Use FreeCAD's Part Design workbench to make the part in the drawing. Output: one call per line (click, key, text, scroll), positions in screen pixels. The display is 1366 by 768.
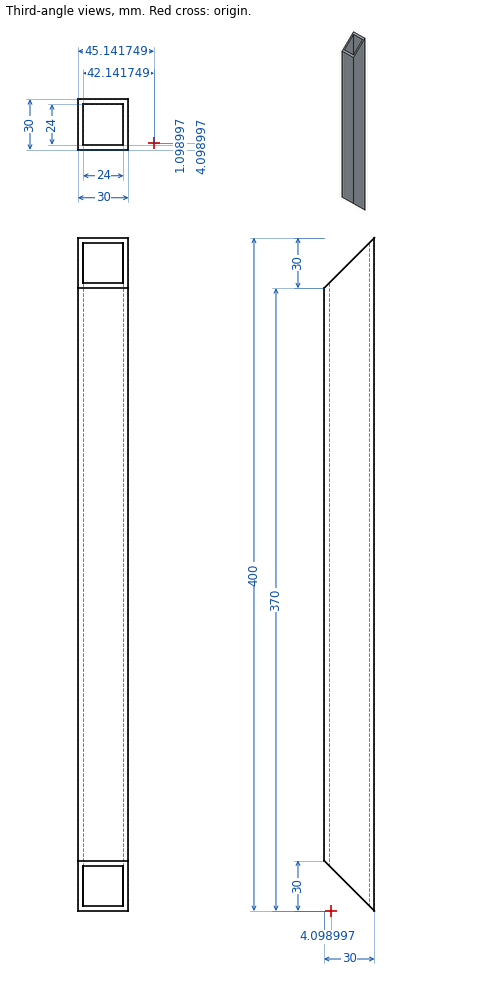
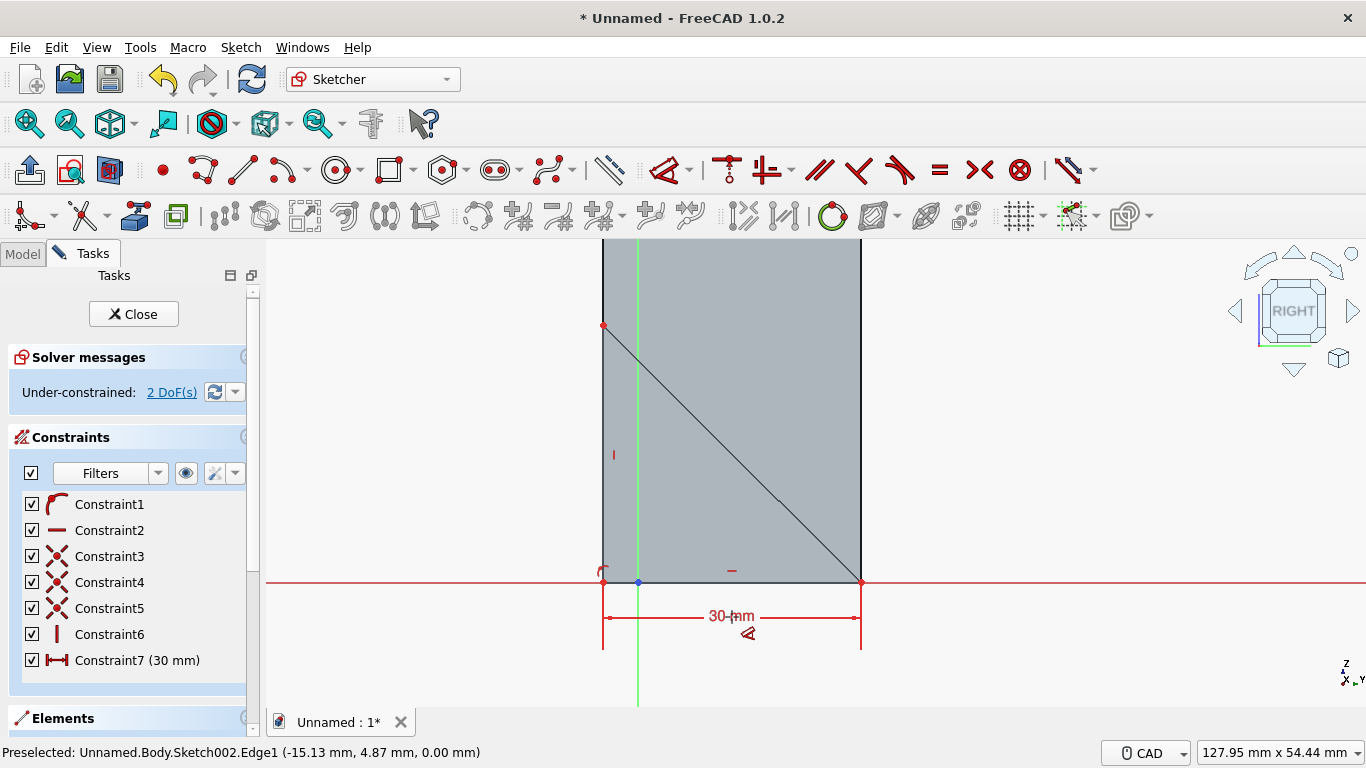
click(603, 403)
click(569, 454)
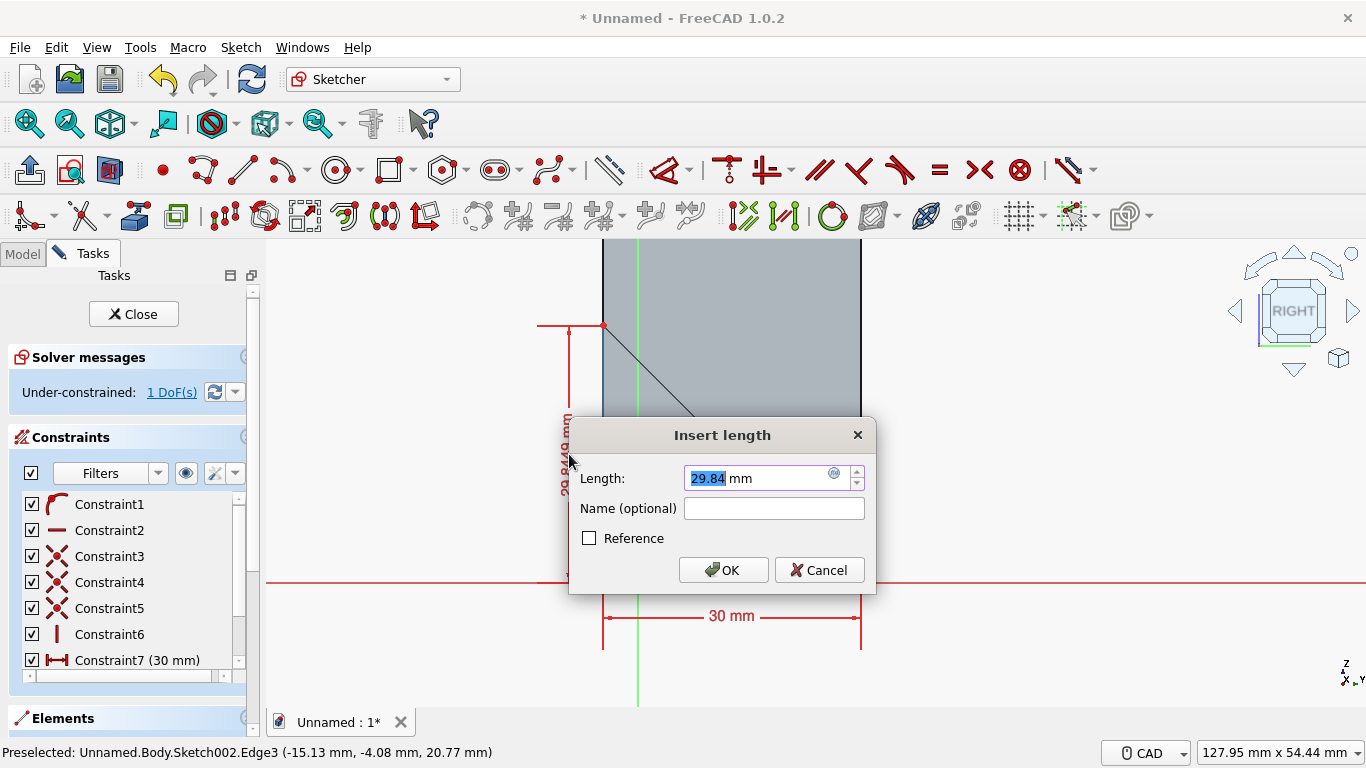
text(30)
key(Return)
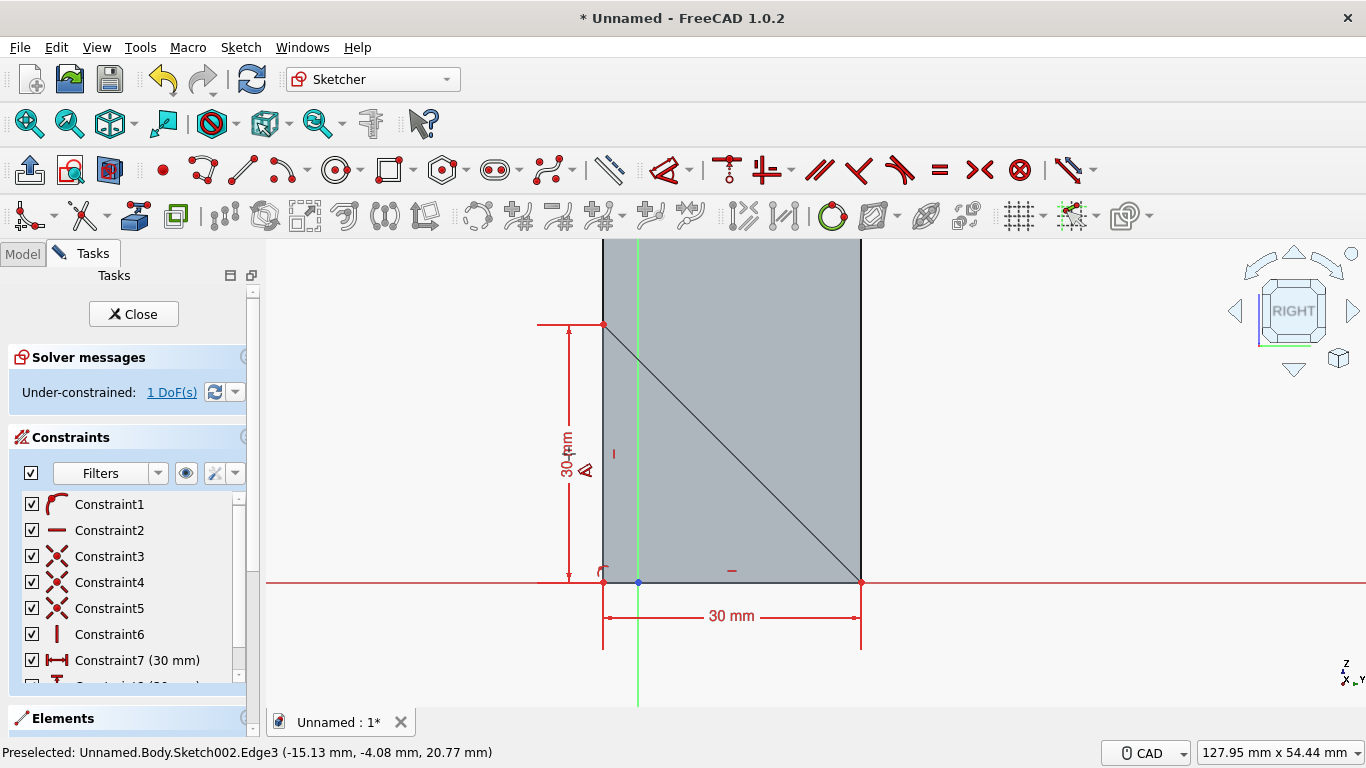
click(603, 583)
click(621, 617)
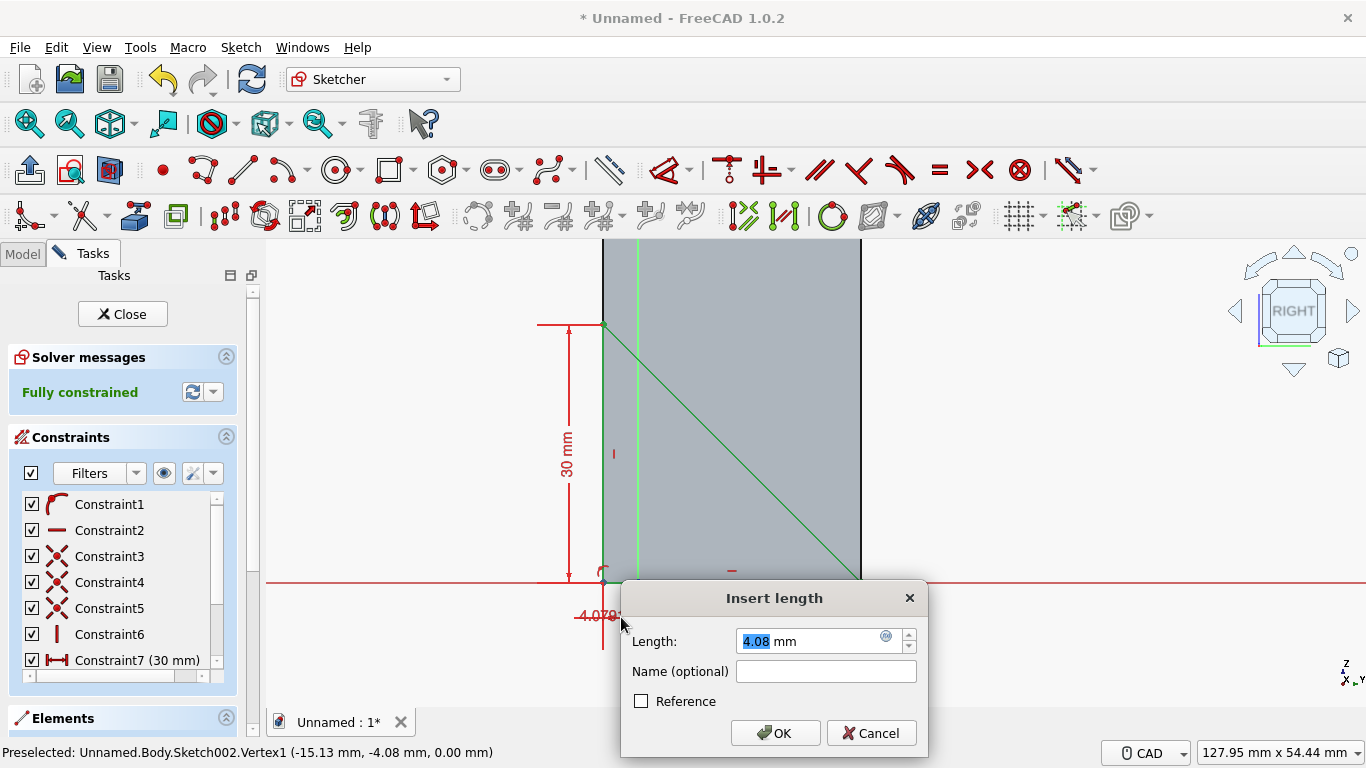
text(4.098997)
key(Return)
key(Escape)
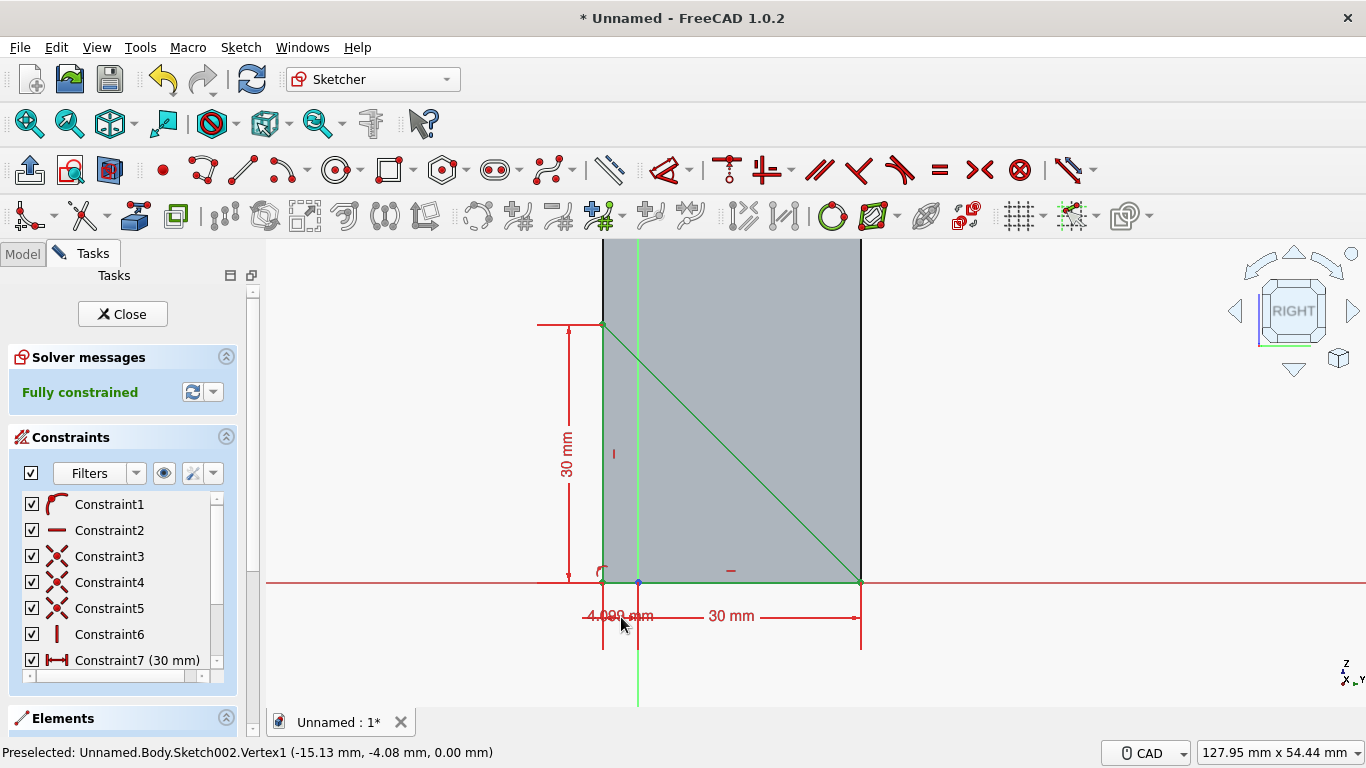
click(123, 314)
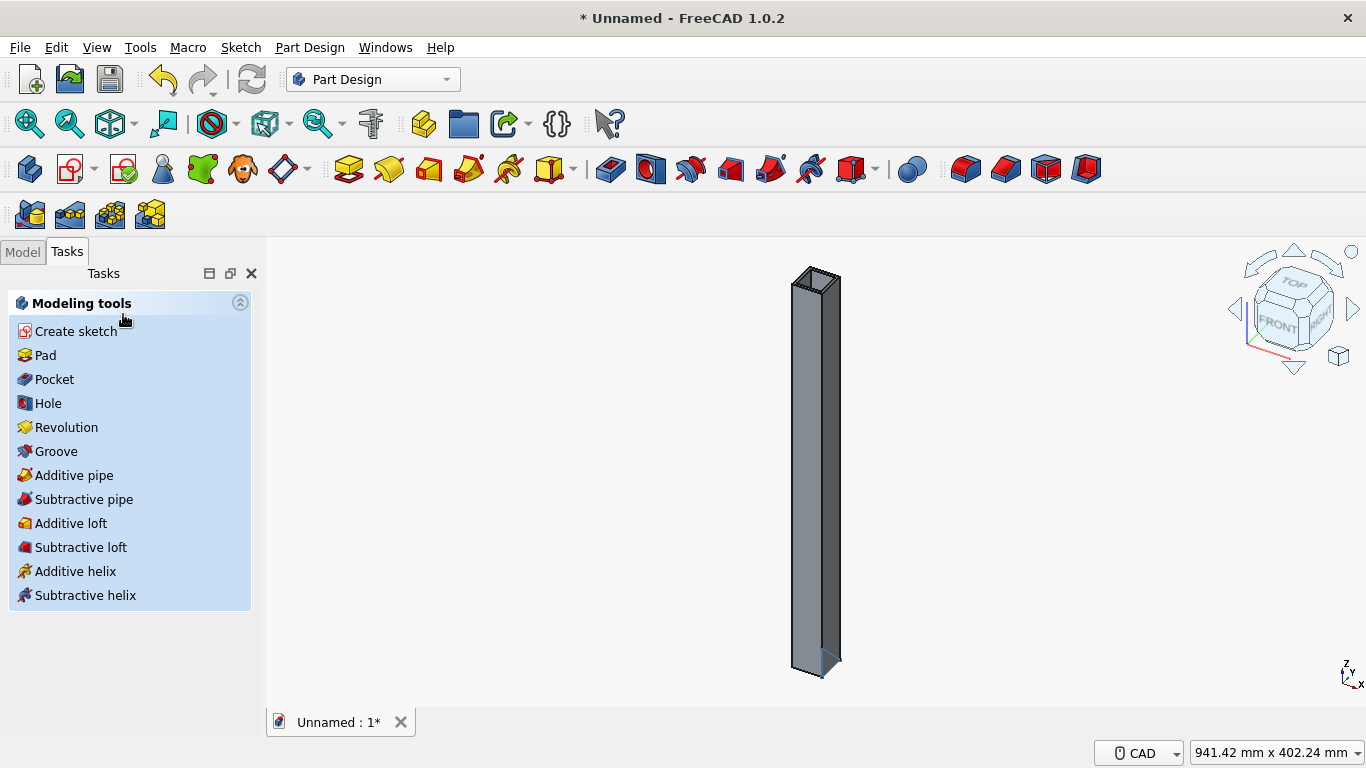
click(612, 170)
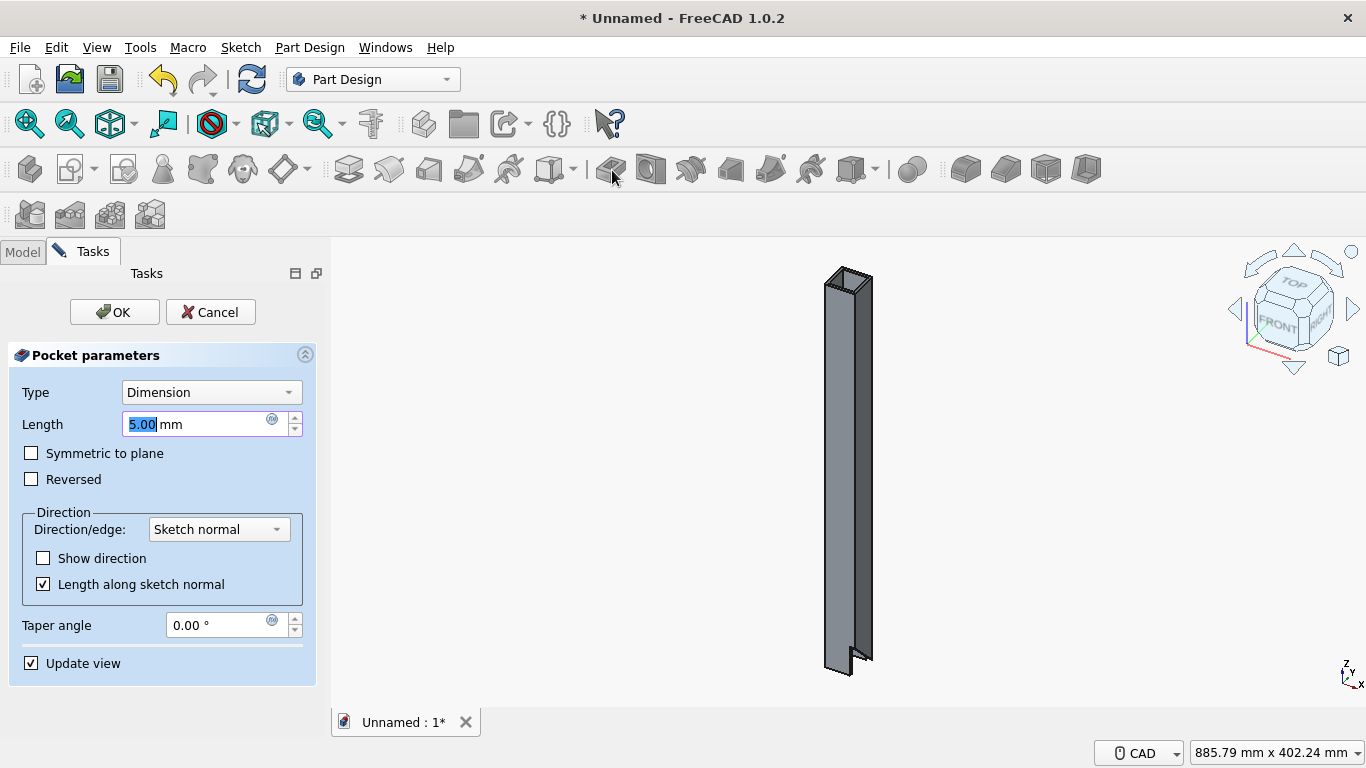
click(212, 392)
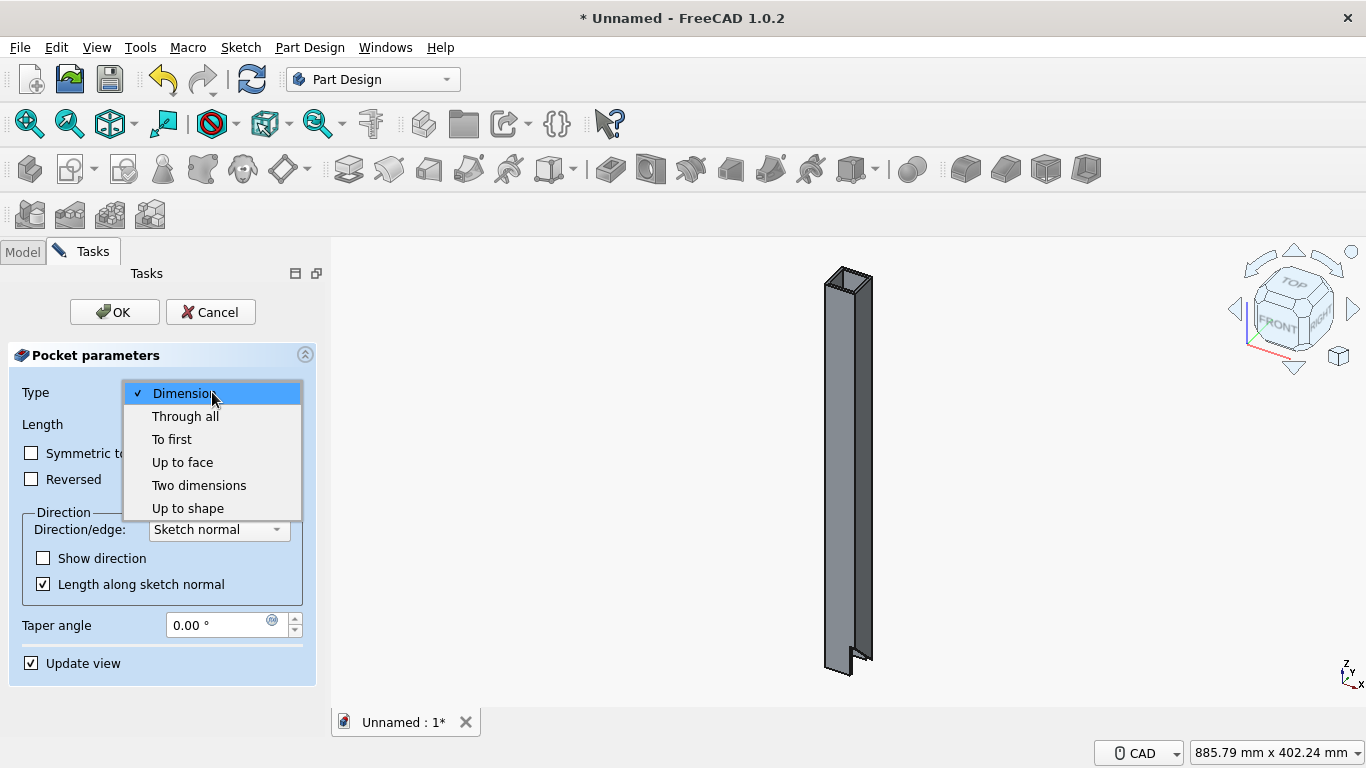
click(212, 416)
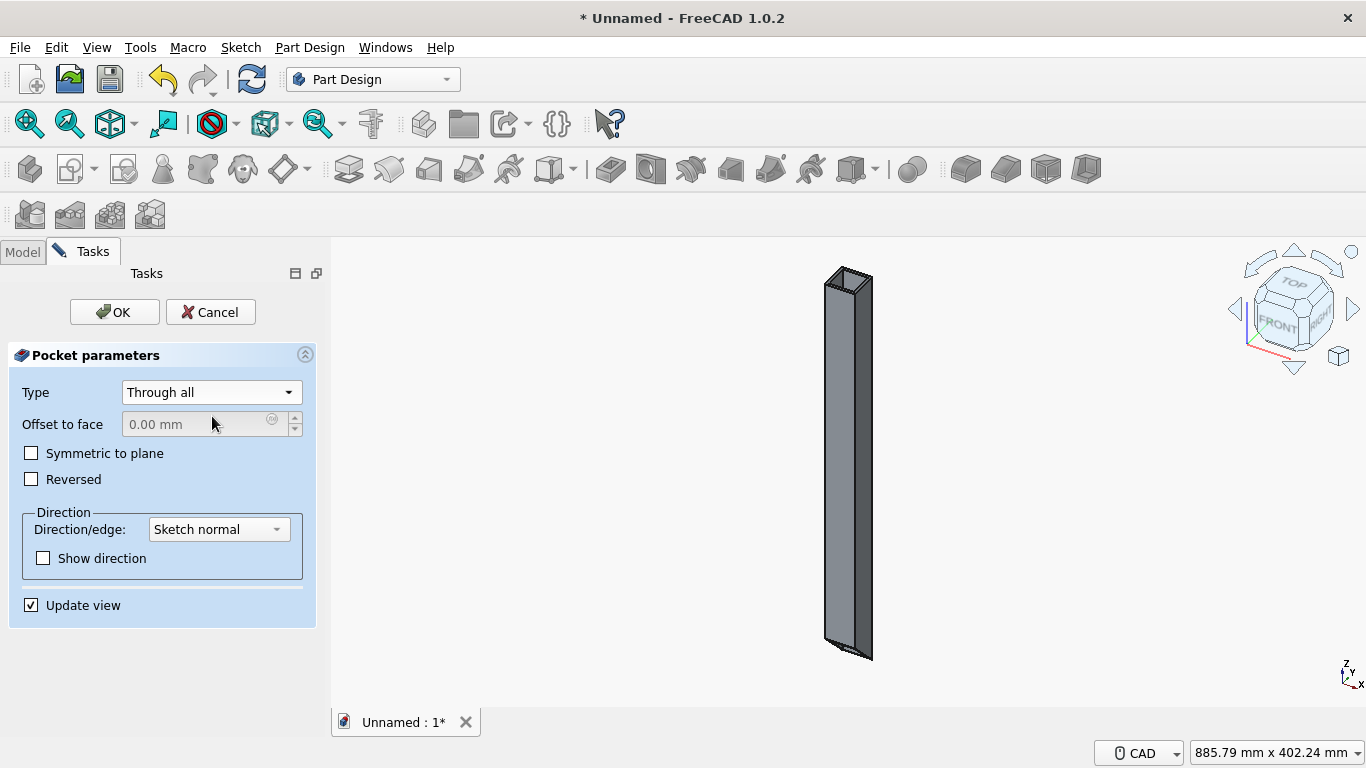
click(115, 312)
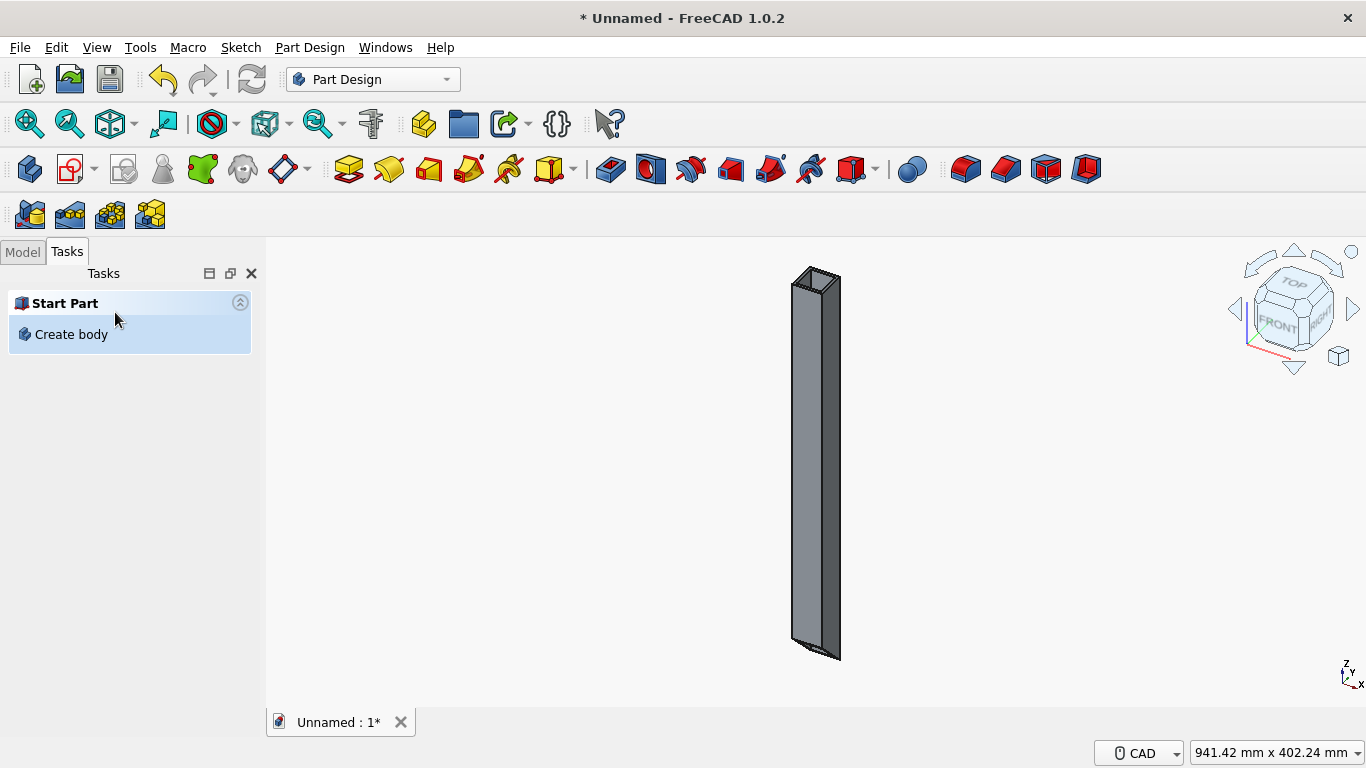
click(831, 312)